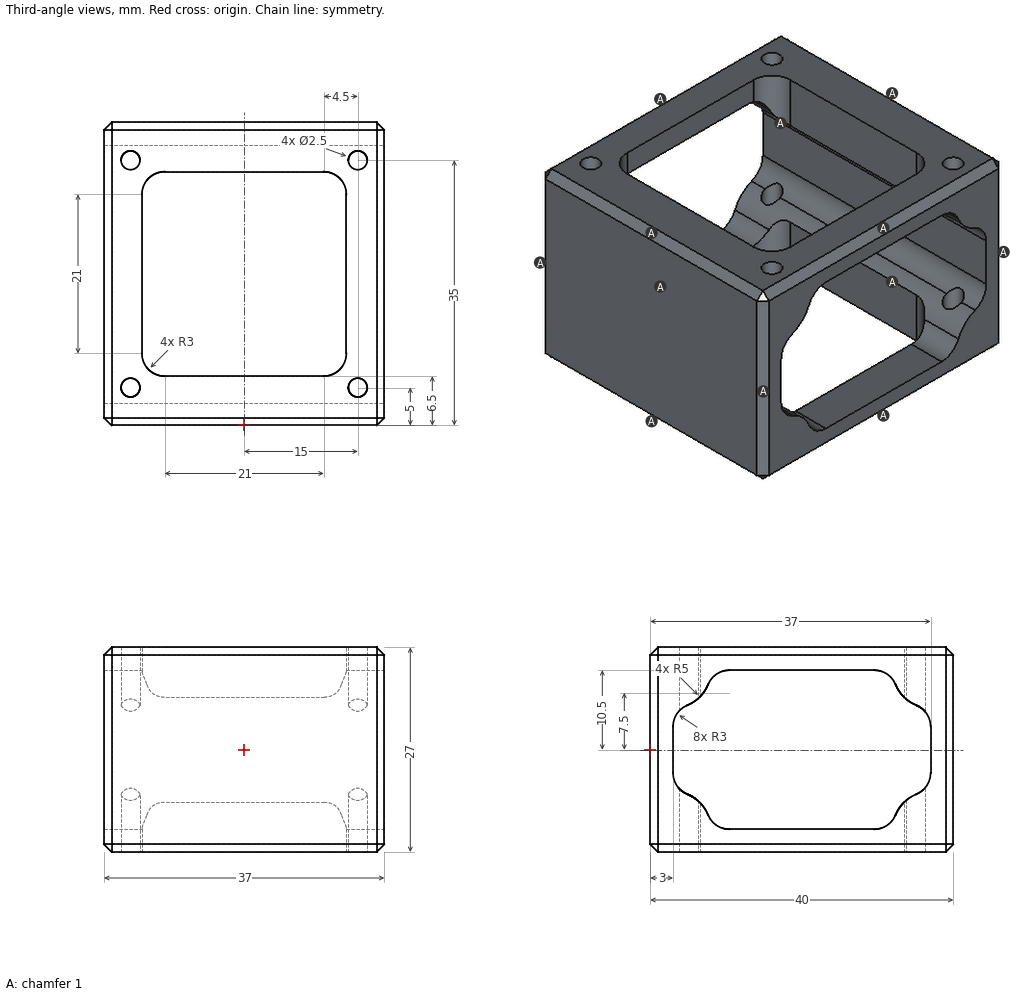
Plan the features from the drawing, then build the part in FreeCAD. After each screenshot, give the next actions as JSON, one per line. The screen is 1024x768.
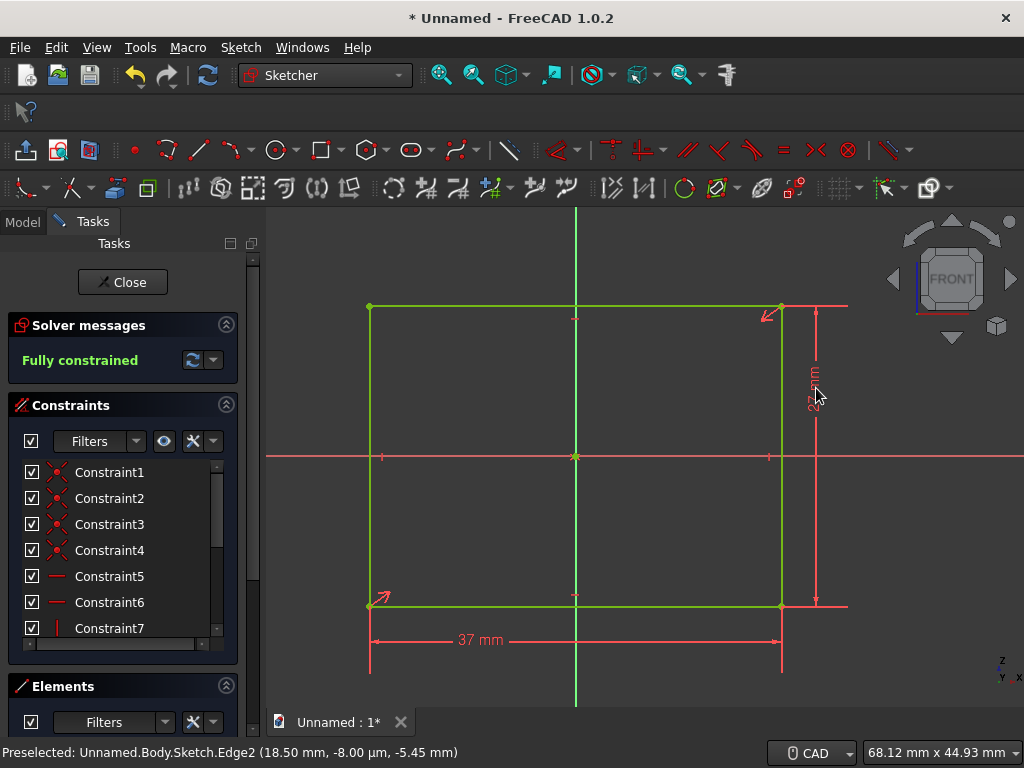
{"action": "left_click", "coordinate": [123, 282]}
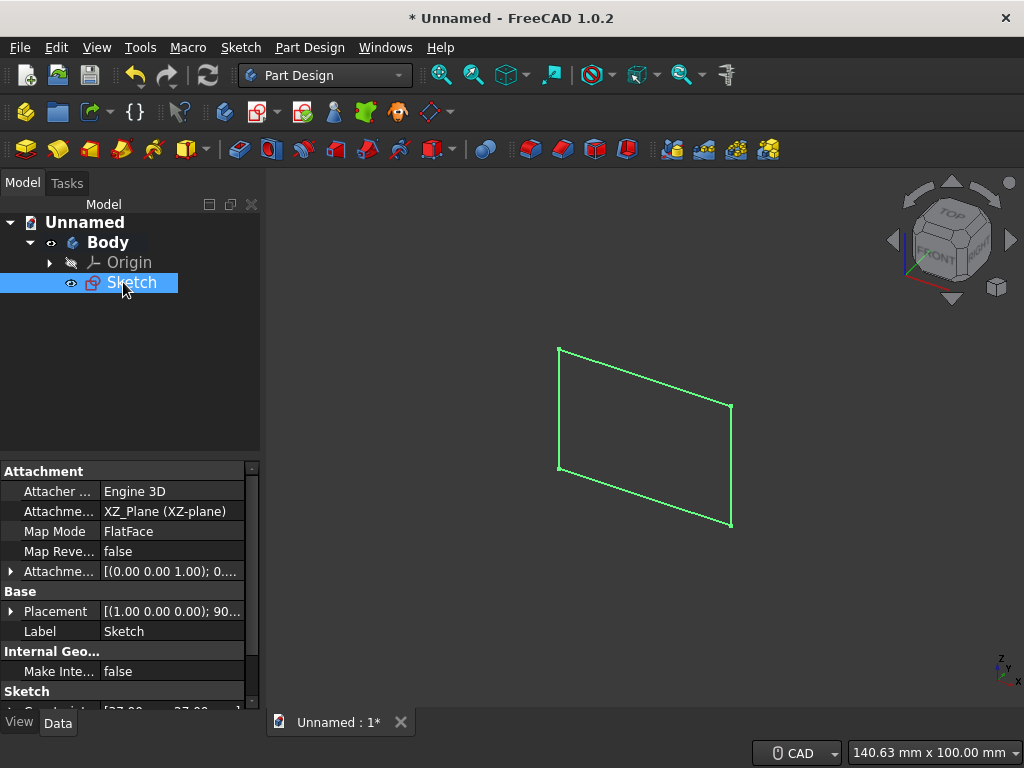
{"action": "left_click", "coordinate": [26, 150]}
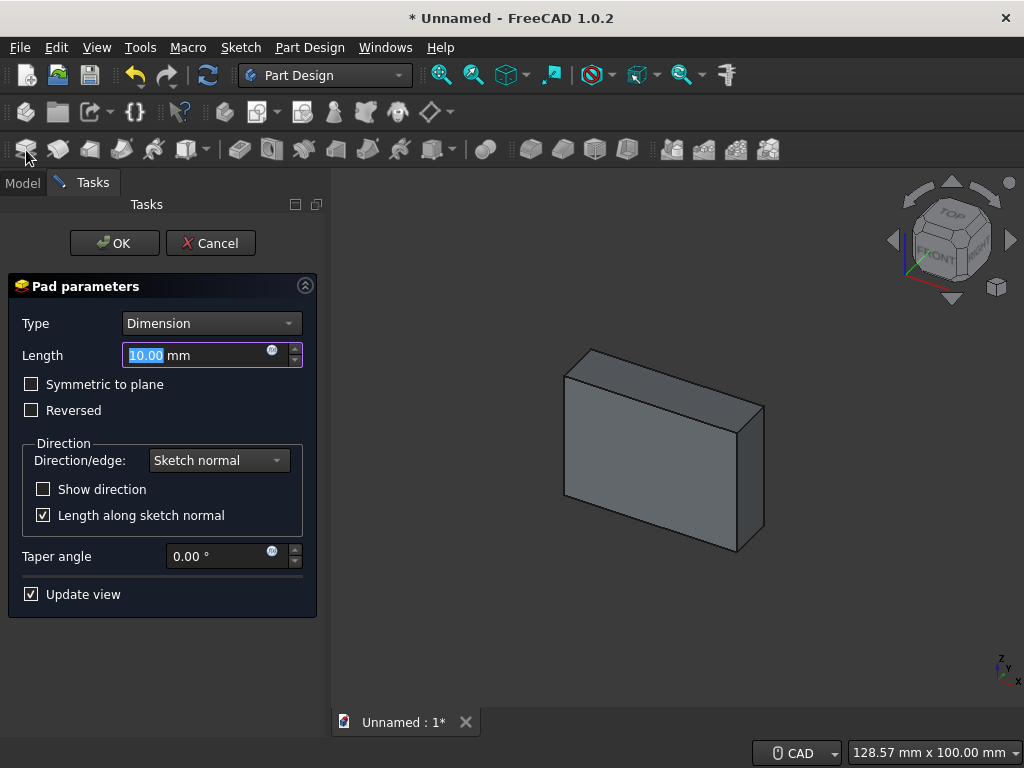
{"action": "type", "text": "40"}
{"action": "key", "text": "Tab"}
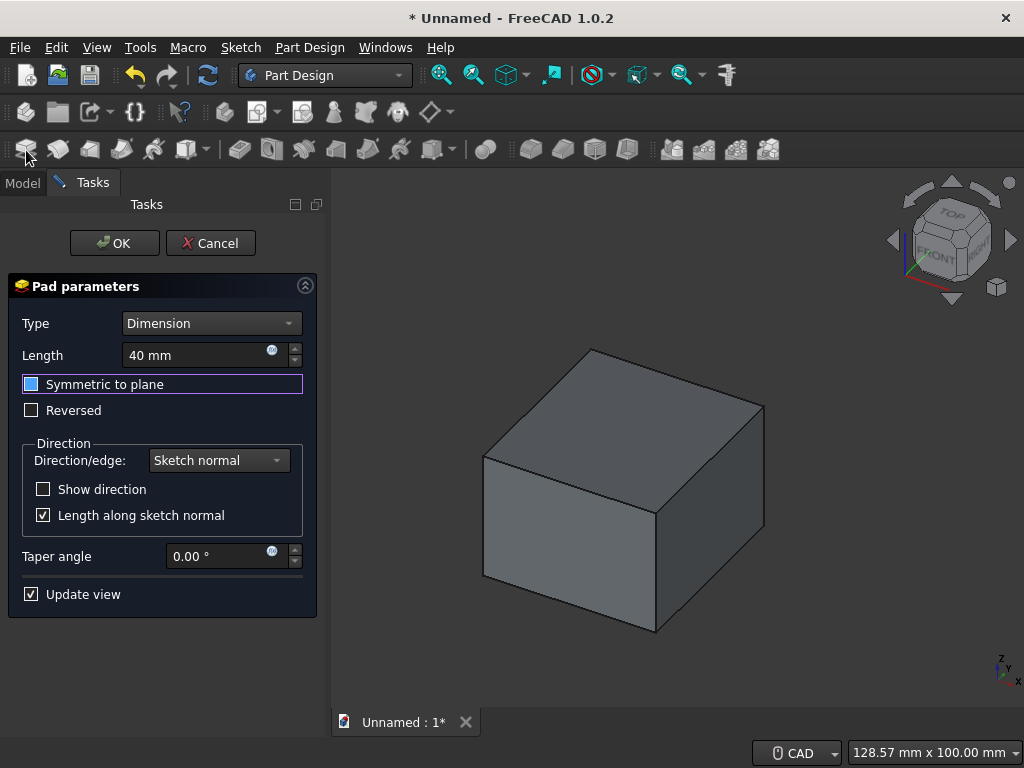
{"action": "left_click", "coordinate": [30, 410]}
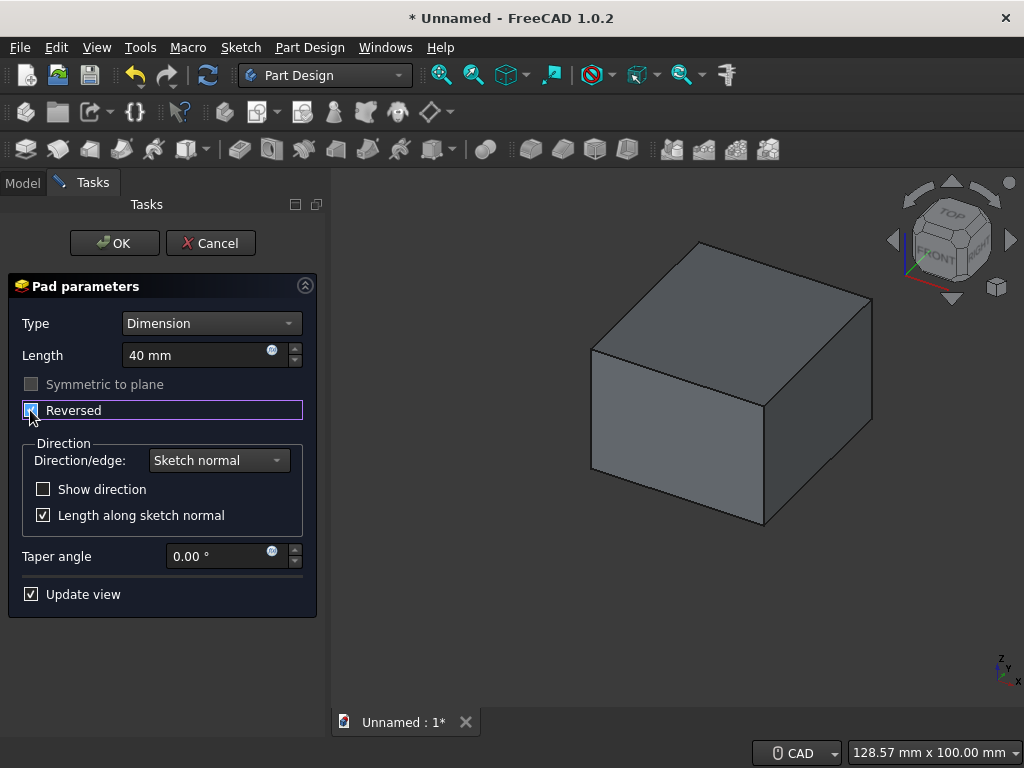
{"action": "left_click", "coordinate": [115, 243]}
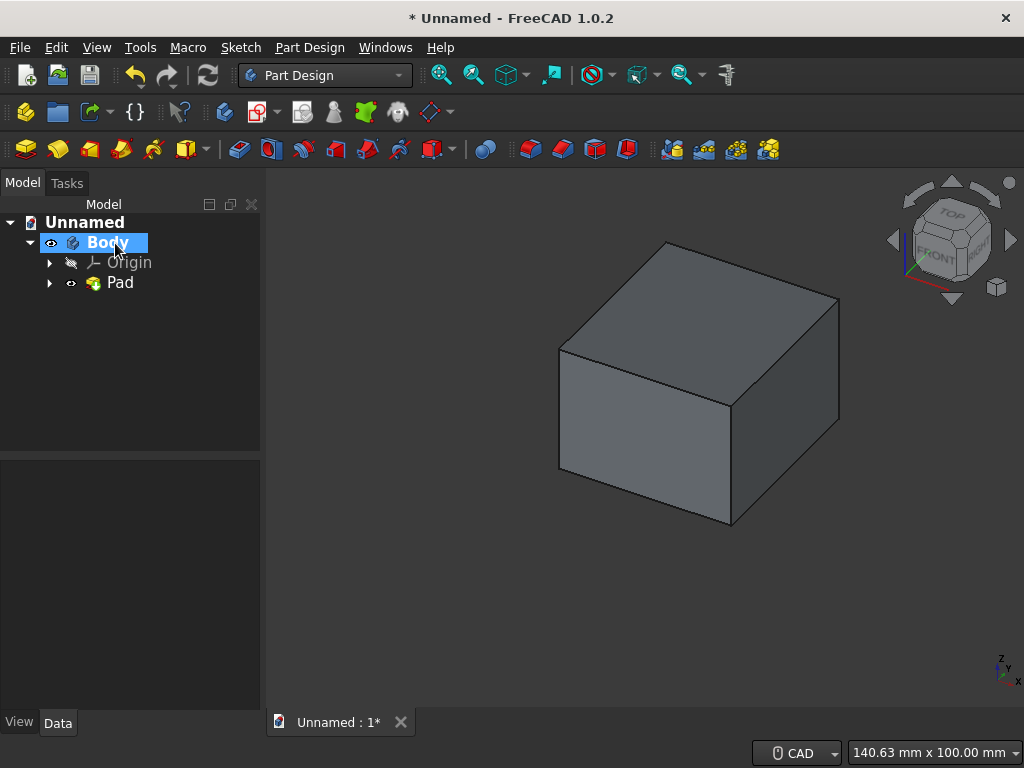
{"action": "key", "text": "5"}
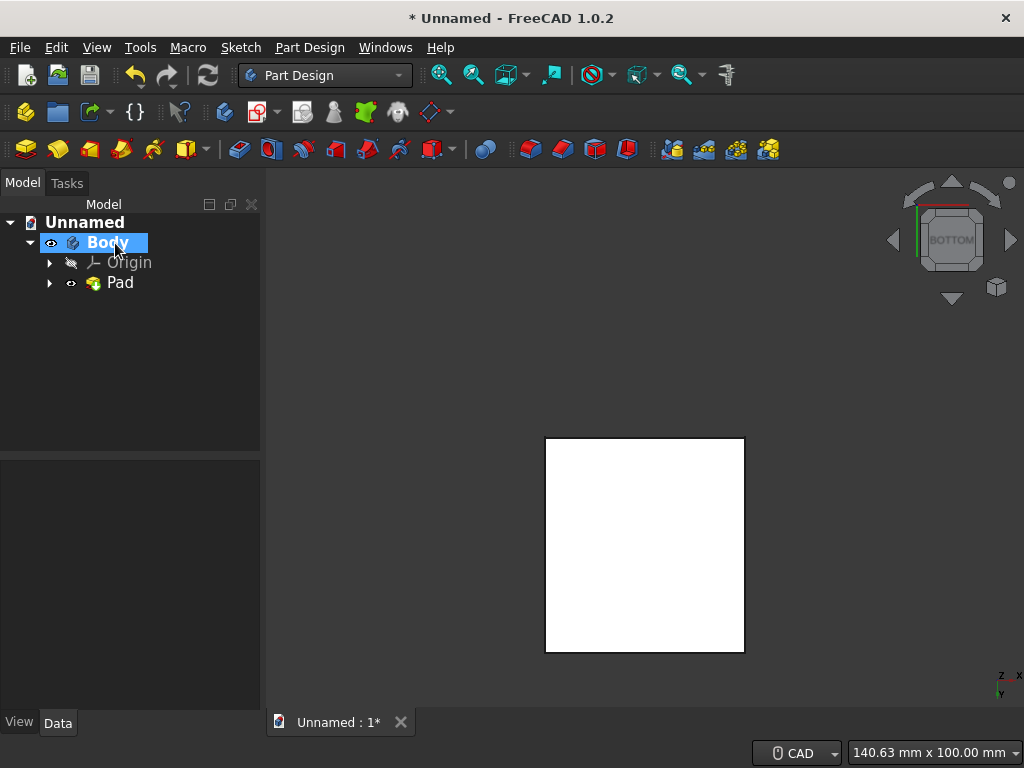
{"action": "key", "text": "v f"}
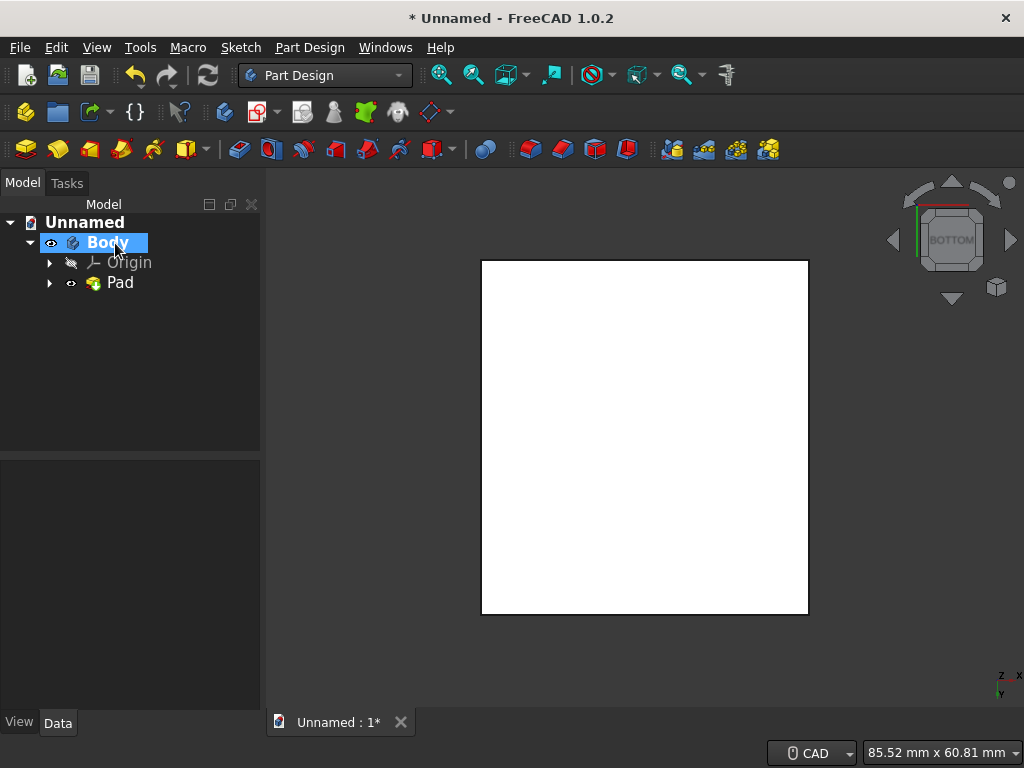
{"action": "left_click", "coordinate": [645, 436]}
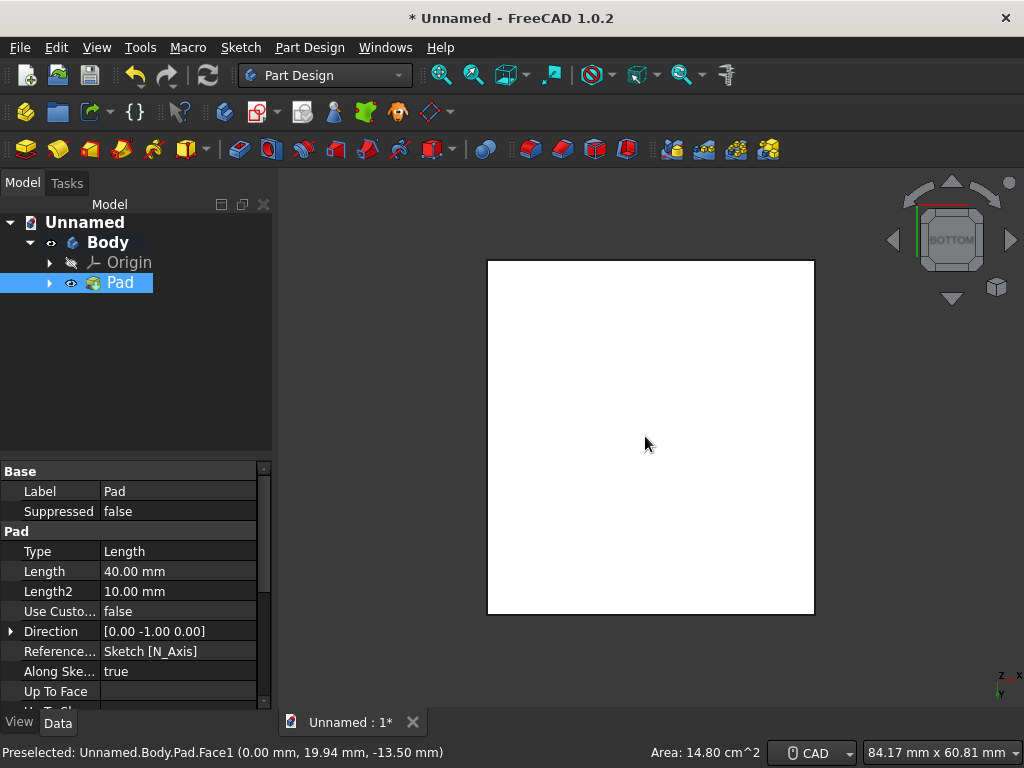
{"action": "left_click", "coordinate": [258, 112]}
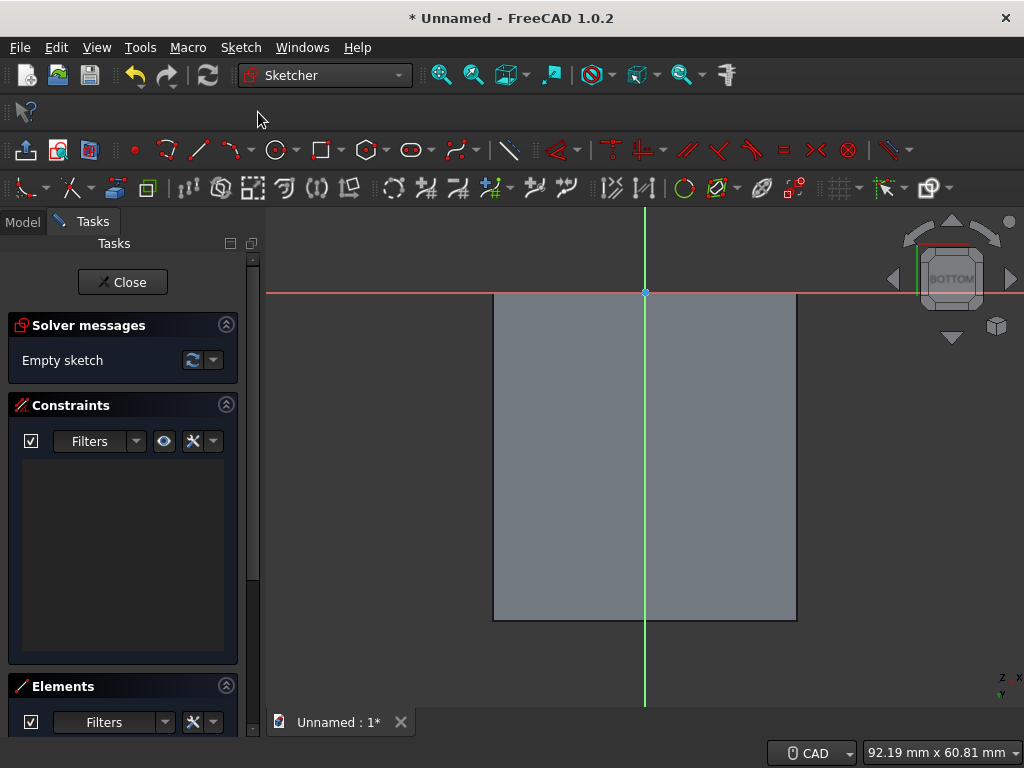
{"action": "key", "text": "g l"}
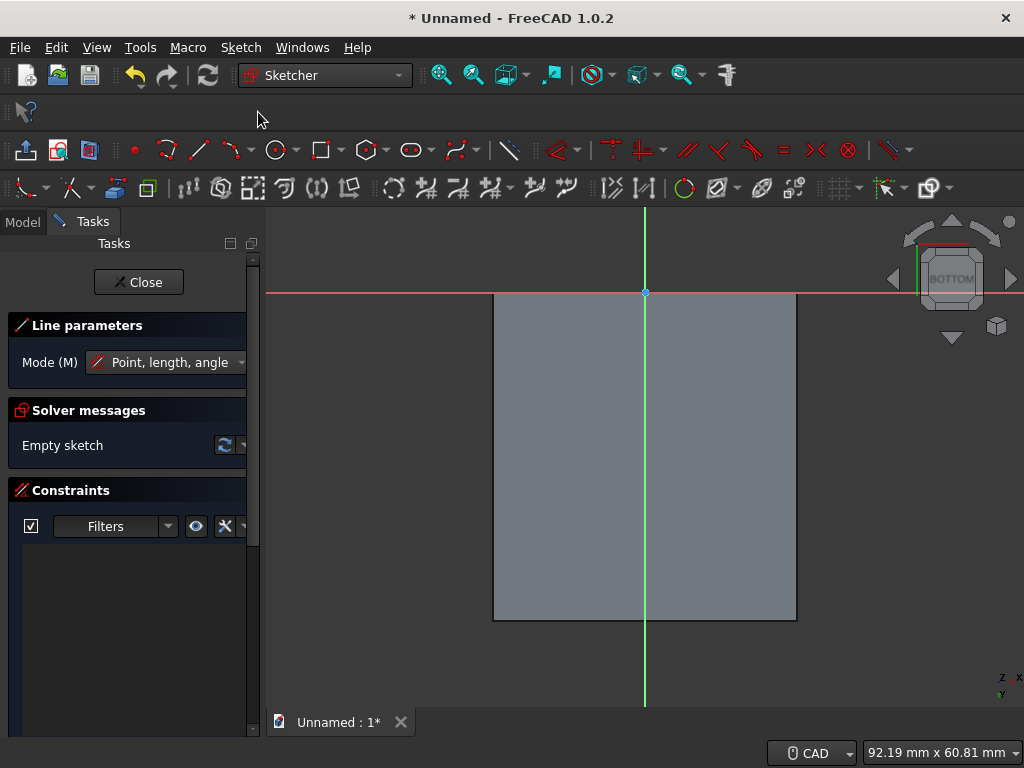
{"action": "left_click", "coordinate": [731, 346]}
{"action": "left_click", "coordinate": [559, 346]}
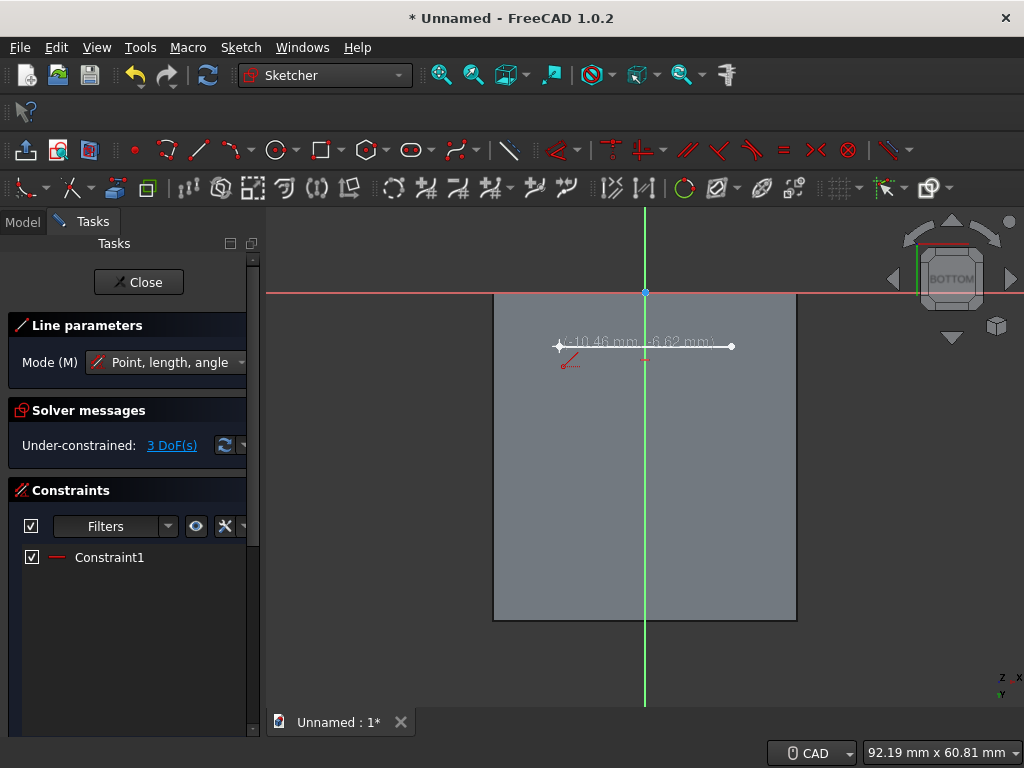
{"action": "left_click", "coordinate": [534, 371]}
{"action": "left_click", "coordinate": [534, 543]}